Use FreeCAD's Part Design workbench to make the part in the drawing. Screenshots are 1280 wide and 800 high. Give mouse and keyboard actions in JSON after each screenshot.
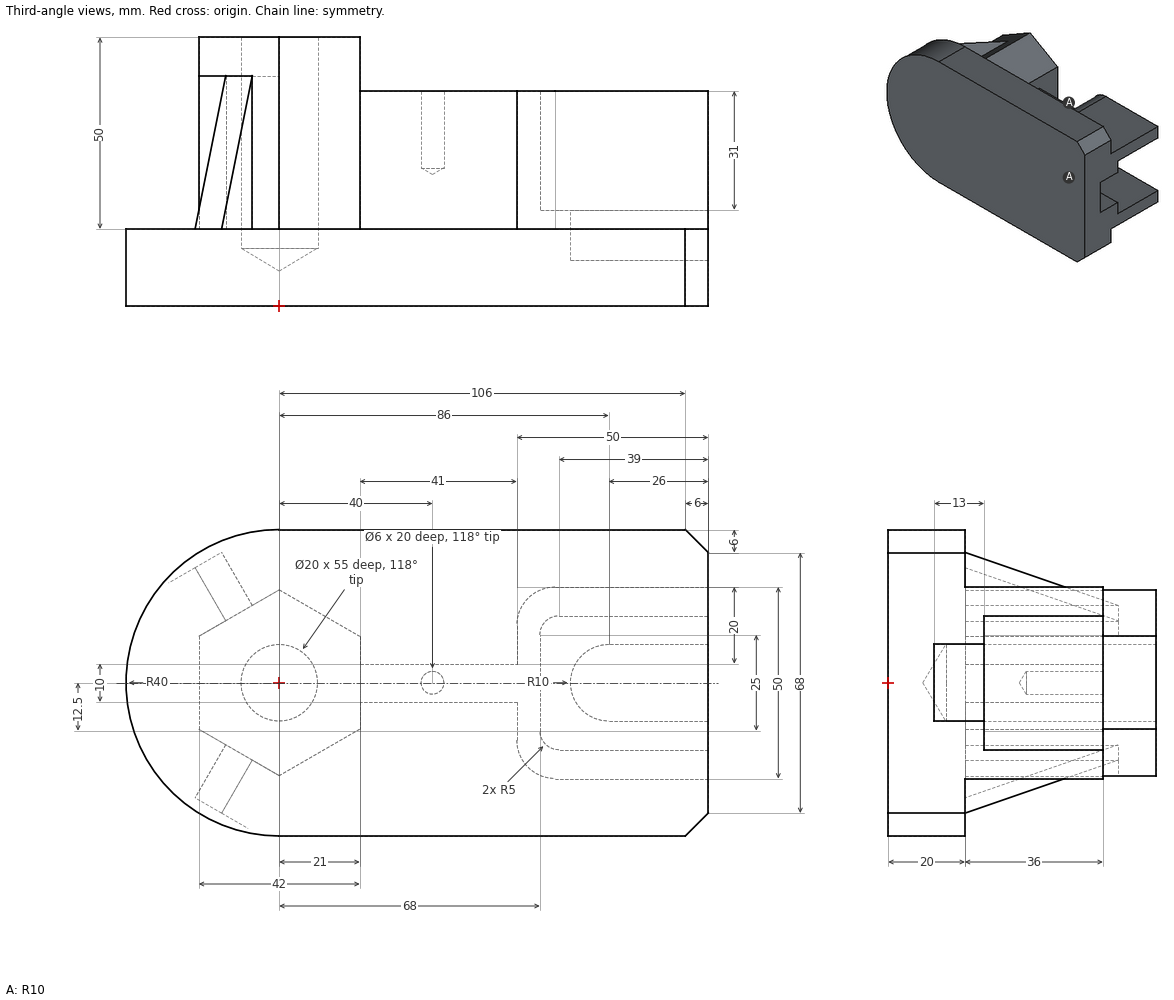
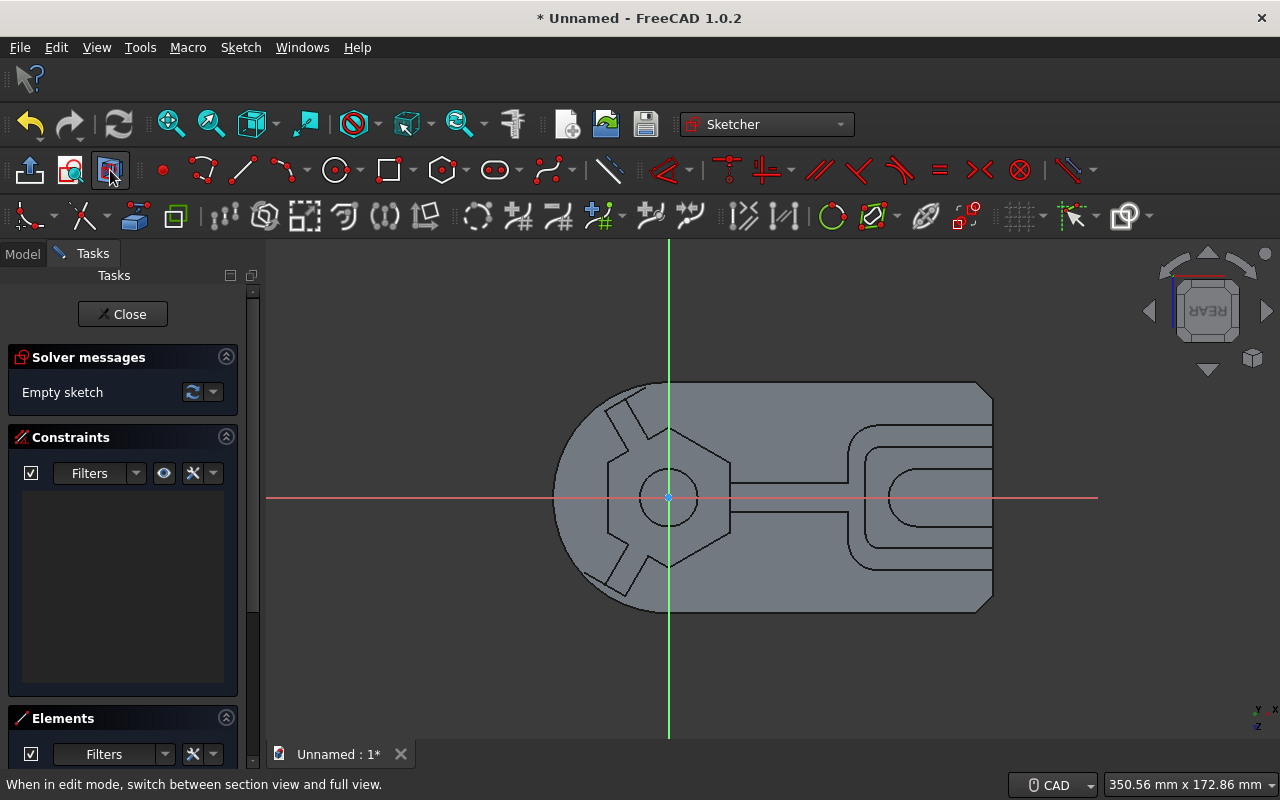
{"action": "scroll", "coordinate": [790, 498], "scroll_direction": "up", "scroll_amount": 14}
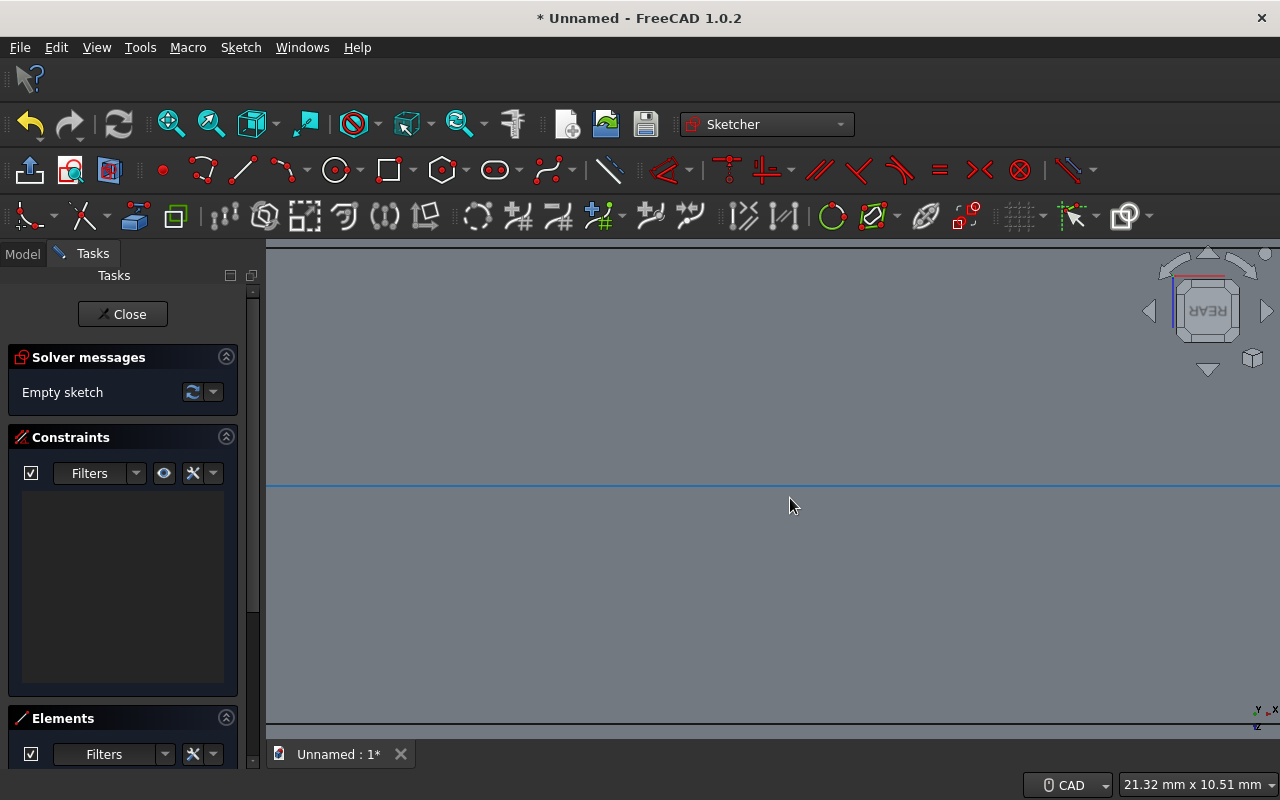
{"action": "left_click", "coordinate": [336, 170]}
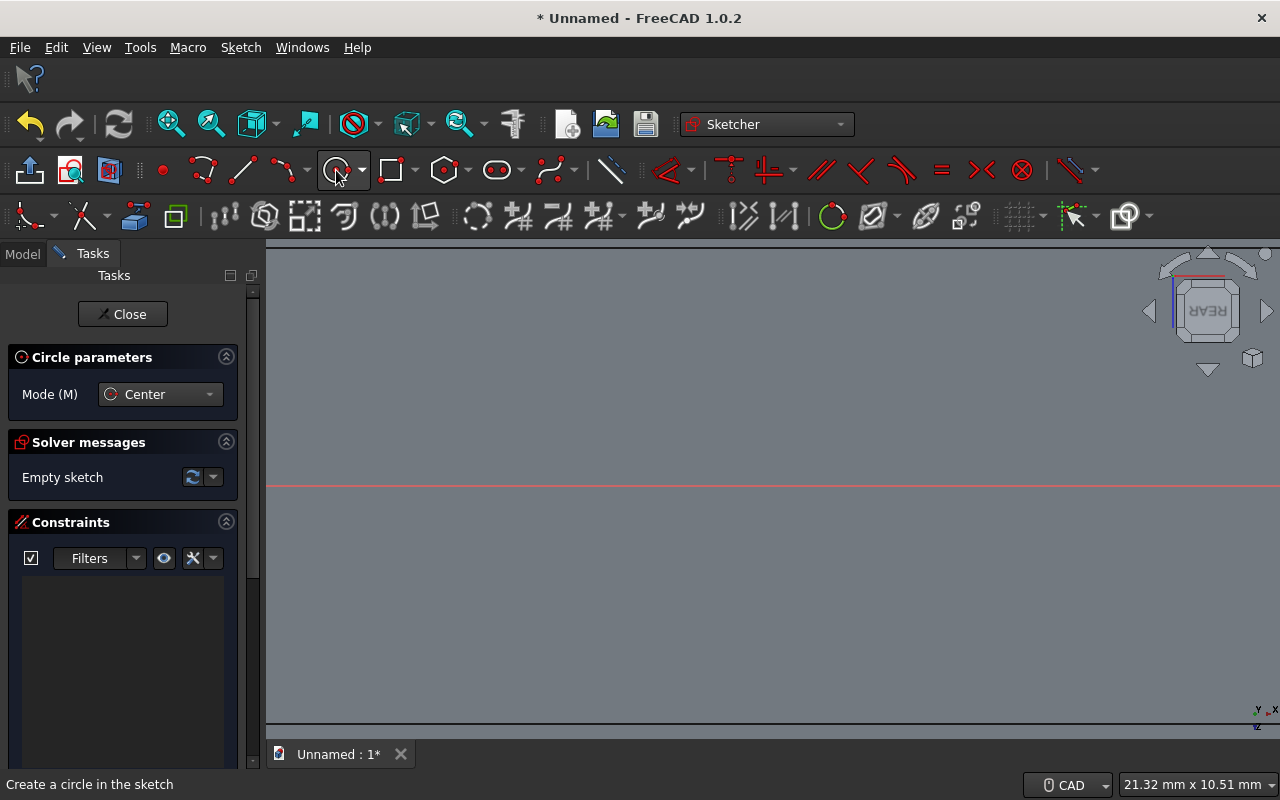
{"action": "left_click", "coordinate": [691, 486]}
{"action": "mouse_move", "coordinate": [792, 385]}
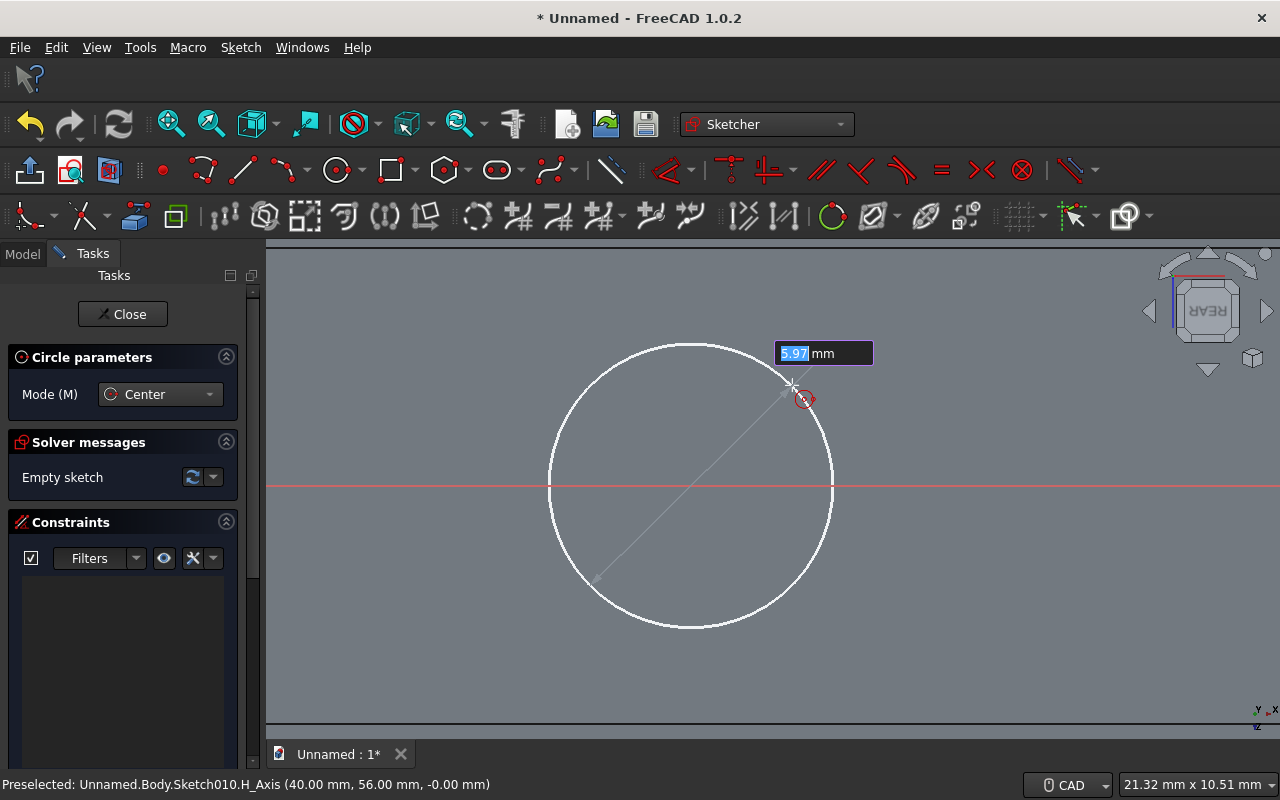
{"action": "type", "text": "6"}
{"action": "key", "text": "Return"}
{"action": "key", "text": "Escape"}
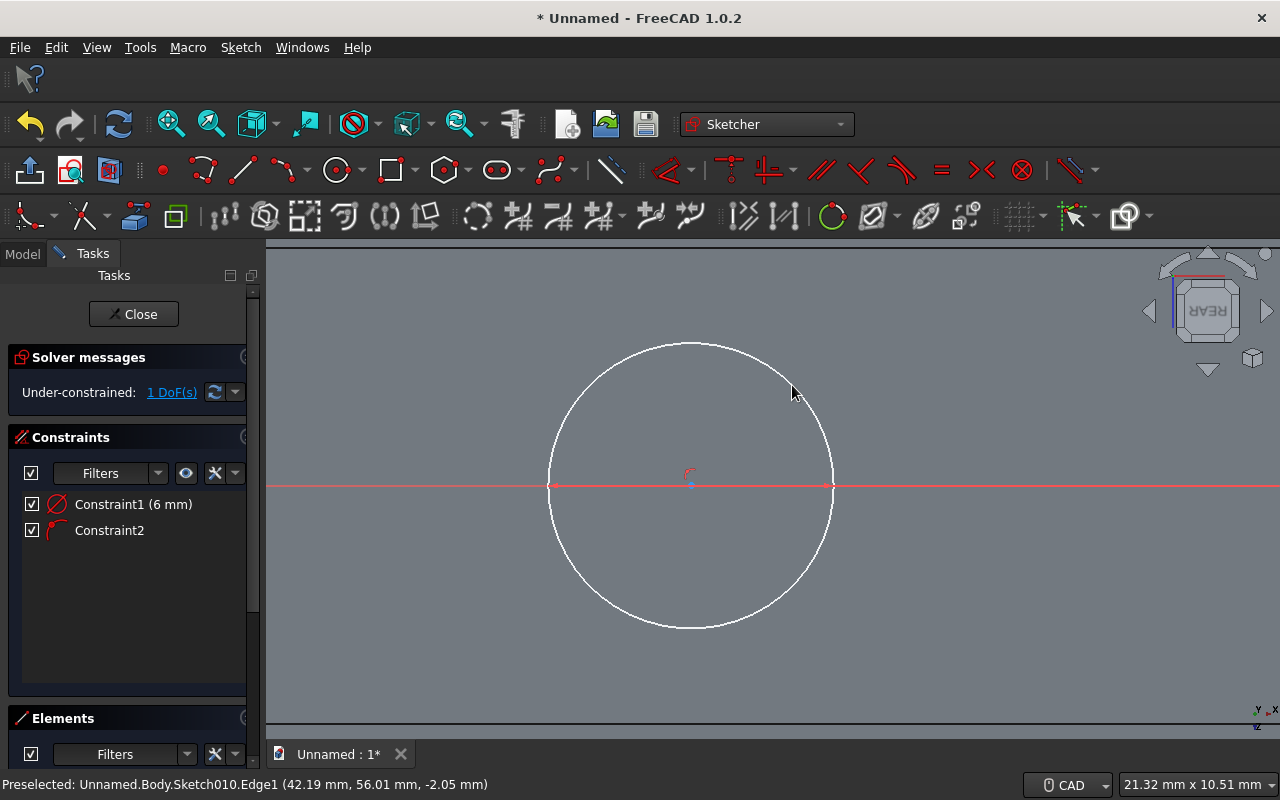
{"action": "left_click", "coordinate": [666, 170]}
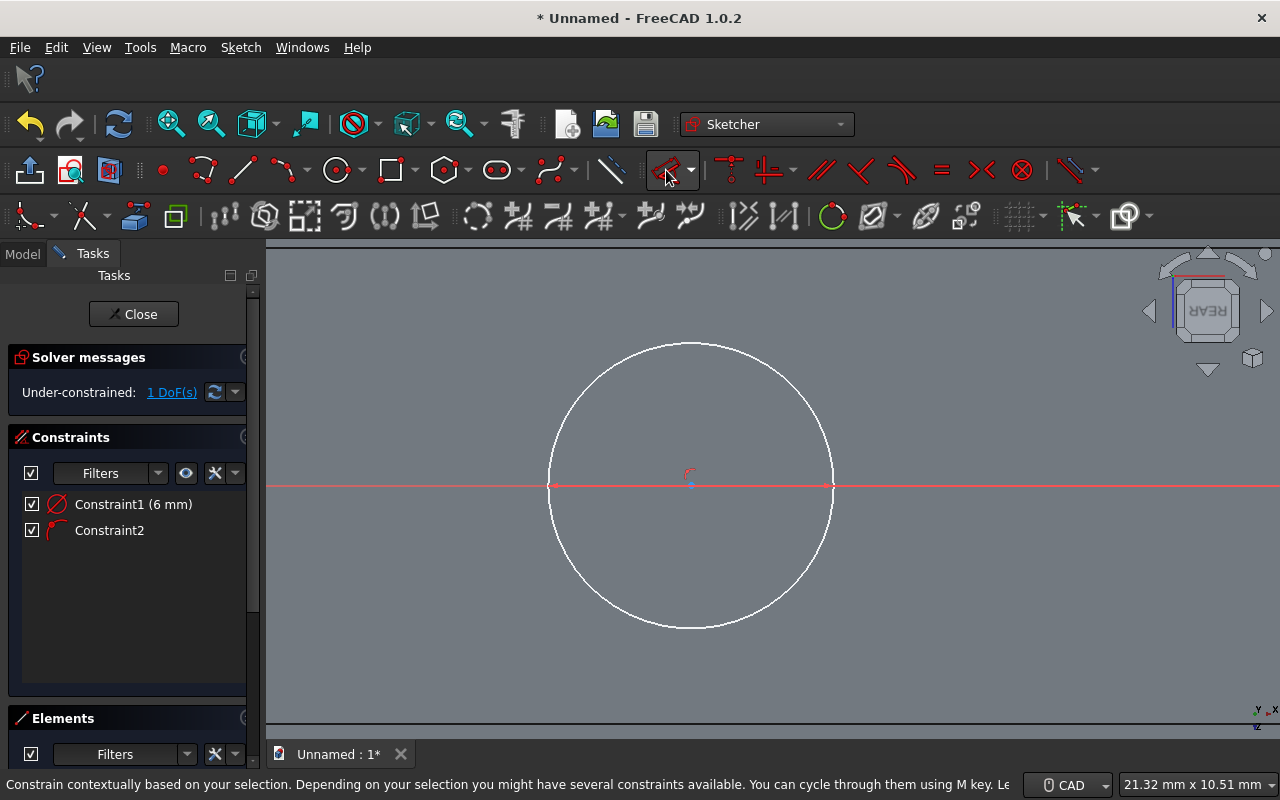
{"action": "left_click", "coordinate": [691, 486]}
{"action": "left_click", "coordinate": [492, 520]}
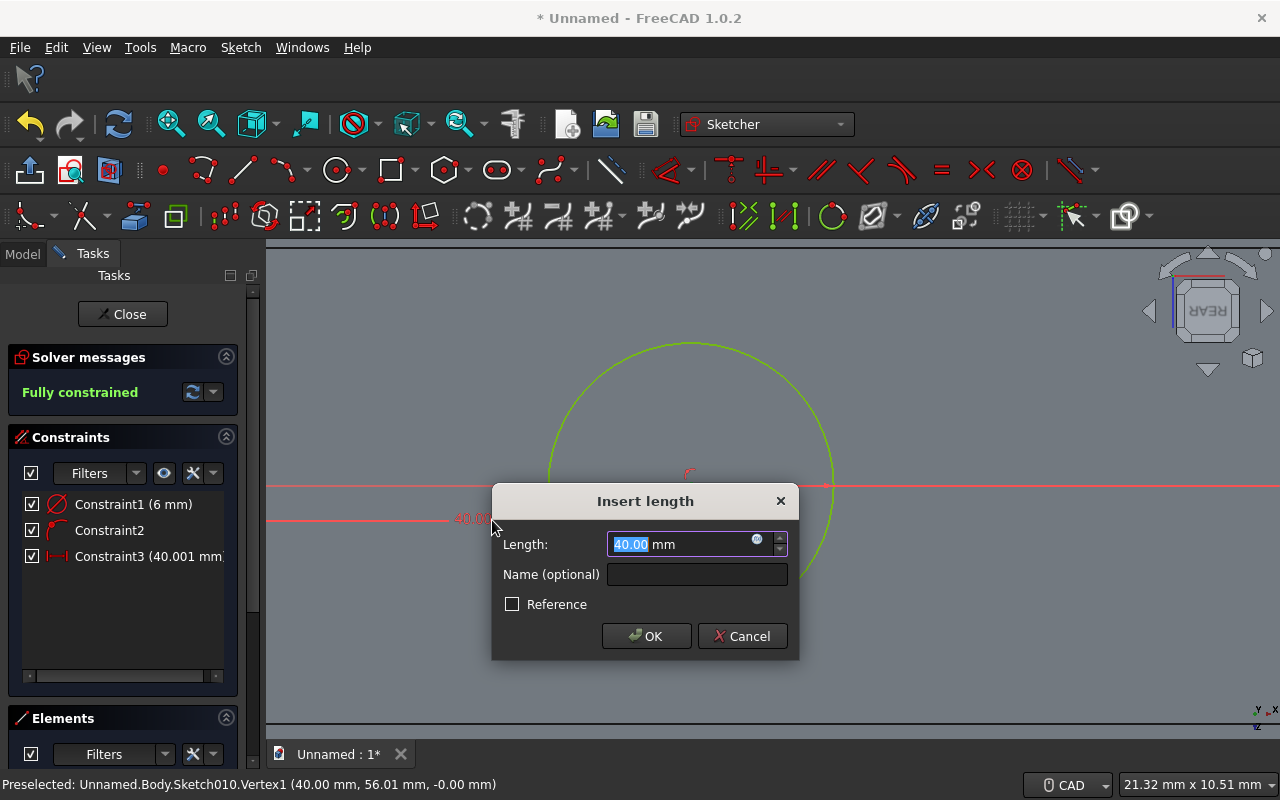
{"action": "type", "text": "40"}
{"action": "key", "text": "Return"}
{"action": "key", "text": "Escape"}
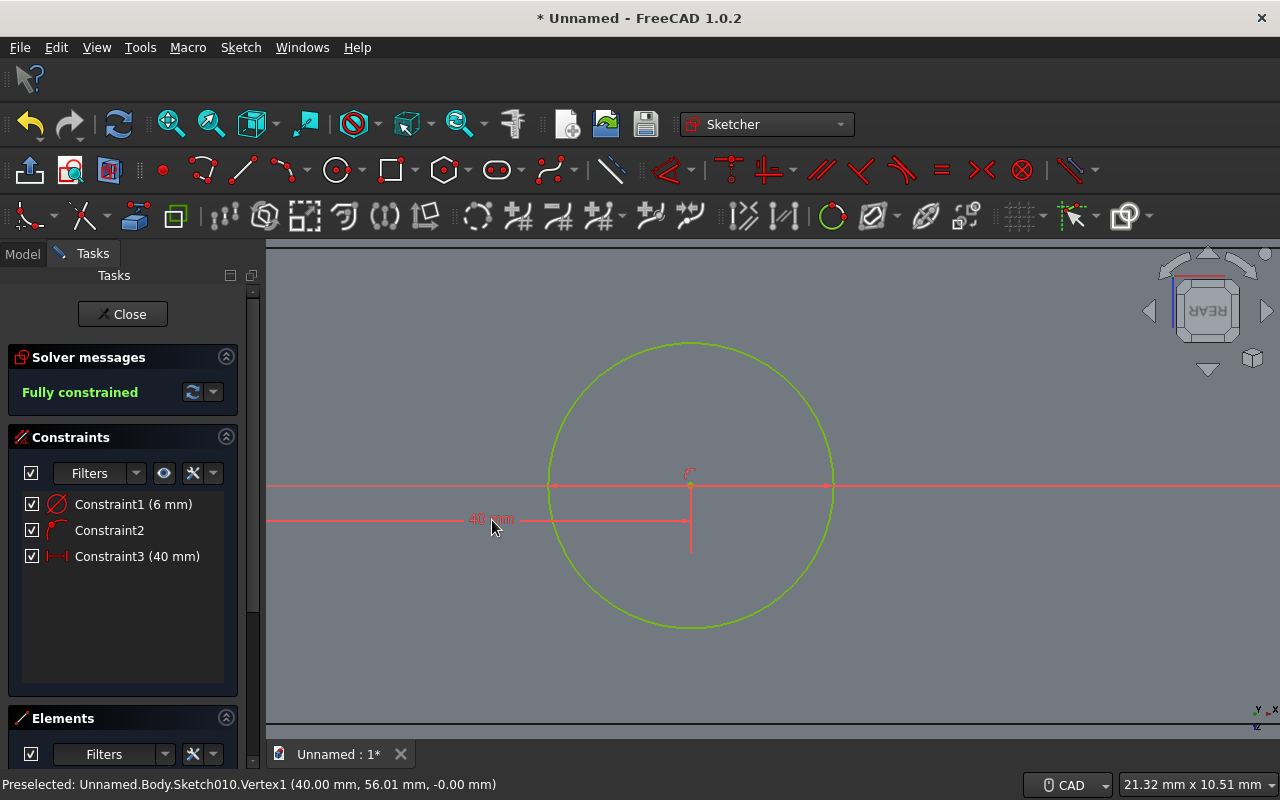
{"action": "left_click", "coordinate": [123, 314]}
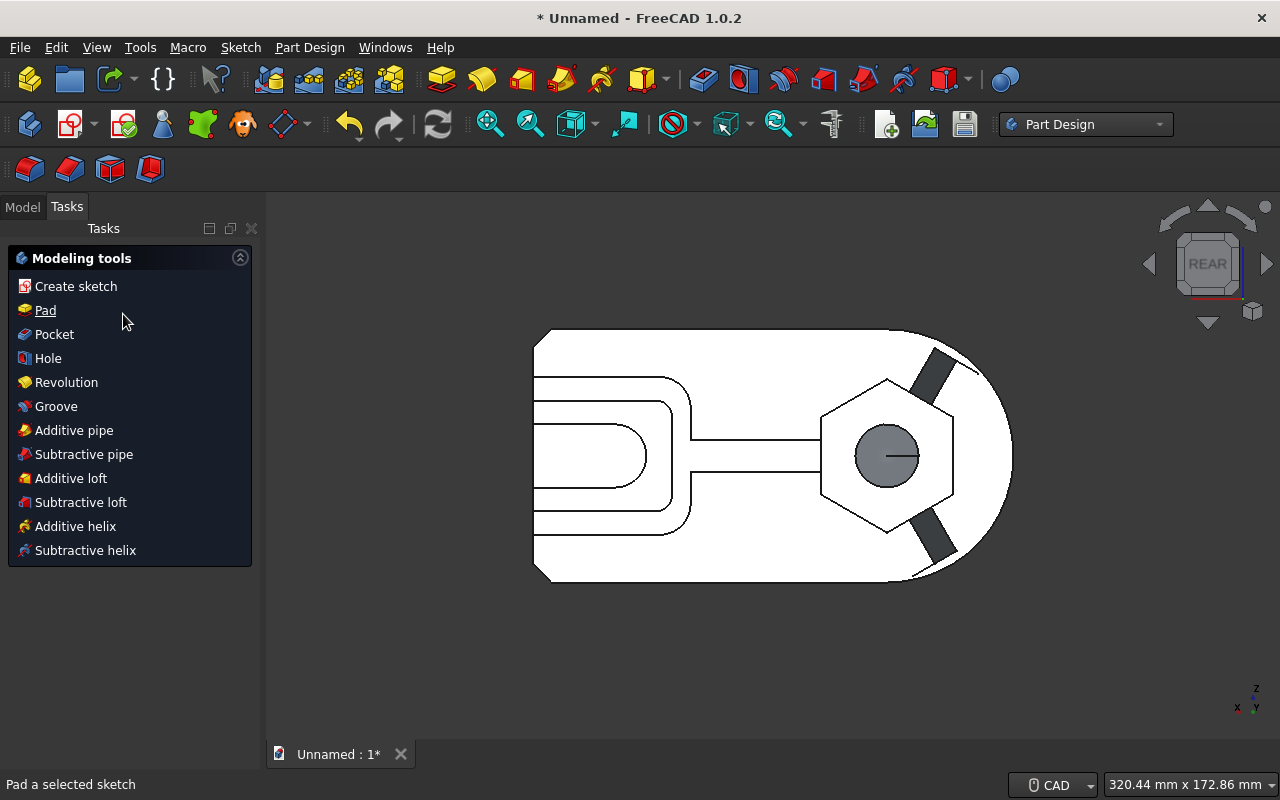
{"action": "left_click", "coordinate": [744, 80]}